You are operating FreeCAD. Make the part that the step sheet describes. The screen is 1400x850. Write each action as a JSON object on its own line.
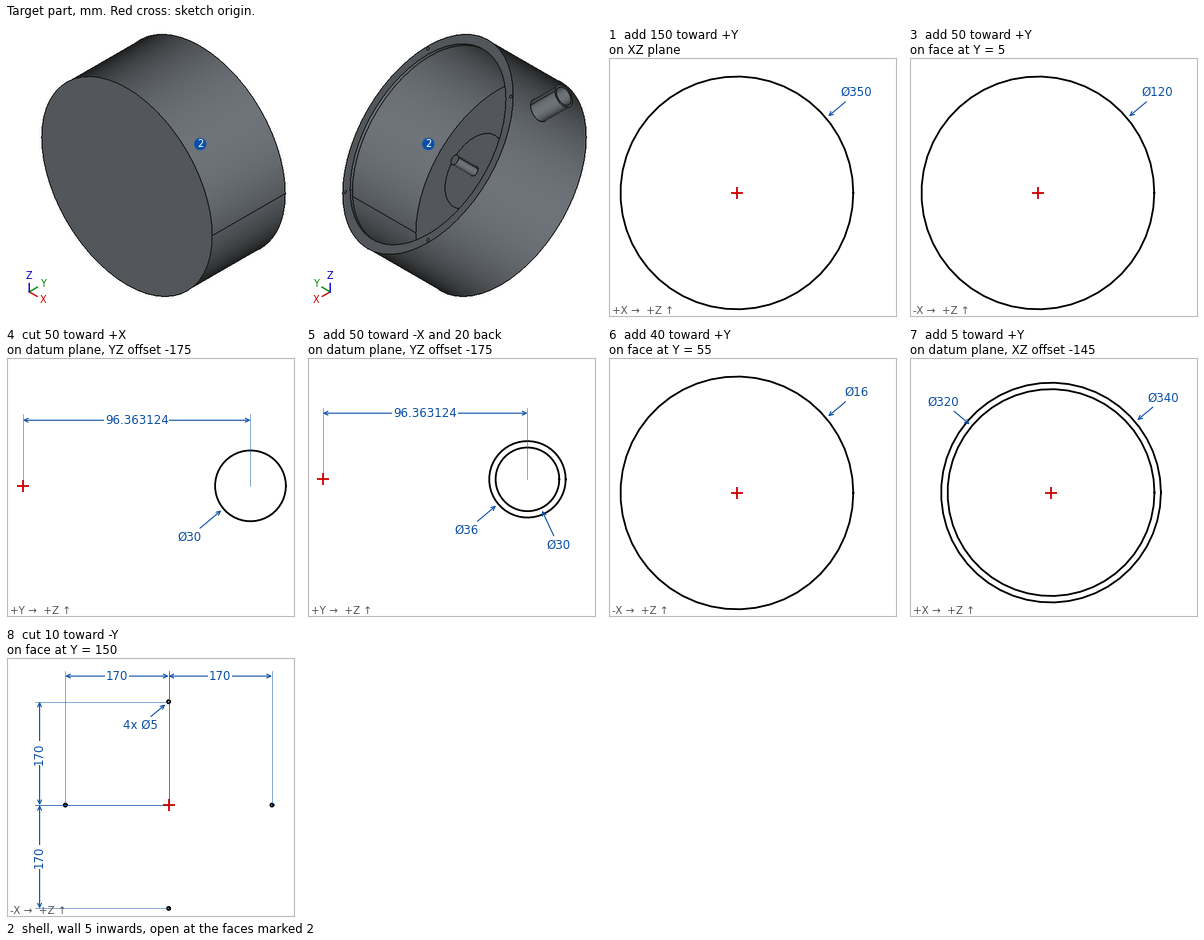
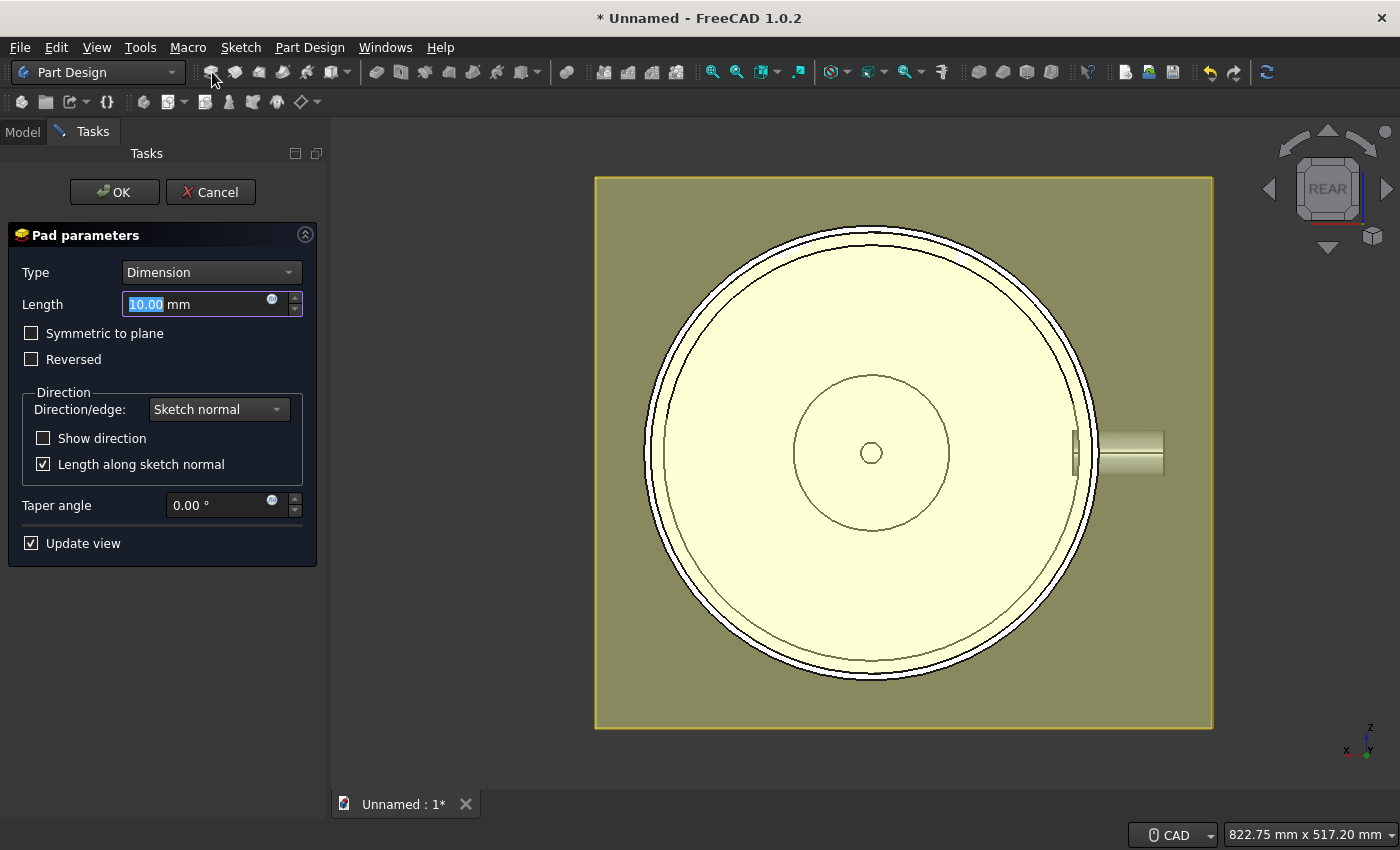
{"action": "type", "text": "5"}
{"action": "key", "text": "Tab"}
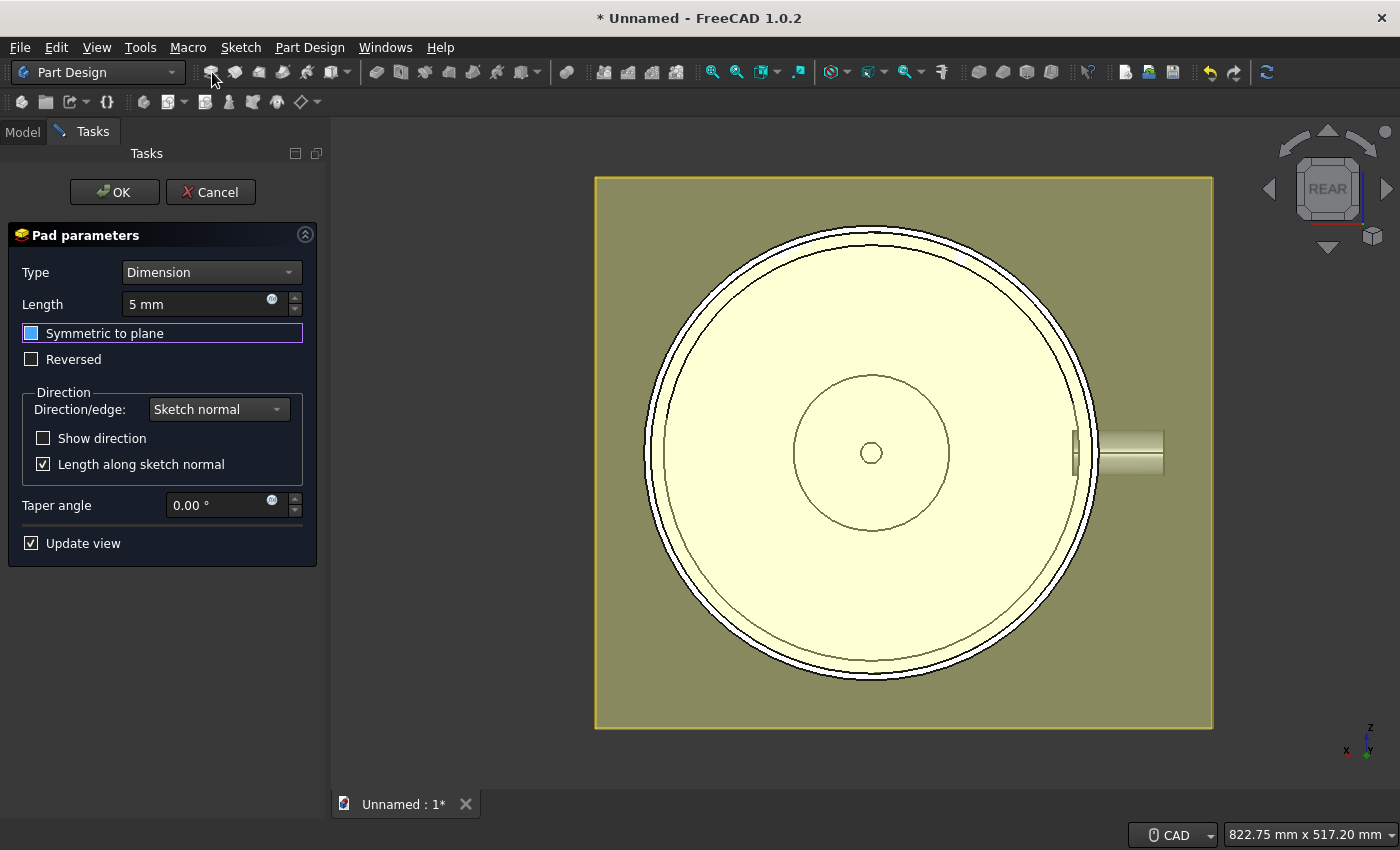
{"action": "left_click", "coordinate": [30, 359]}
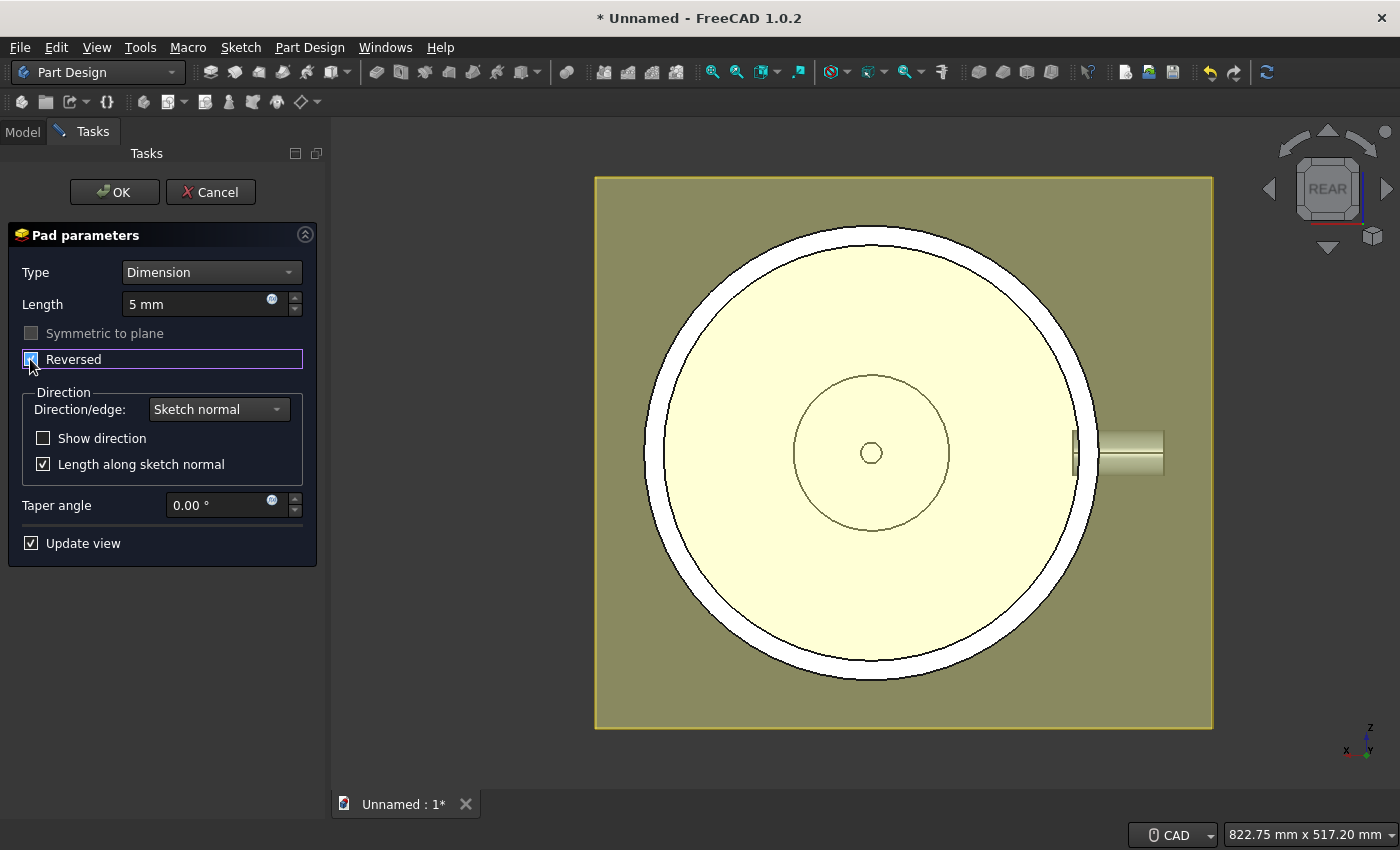
{"action": "left_click", "coordinate": [115, 192]}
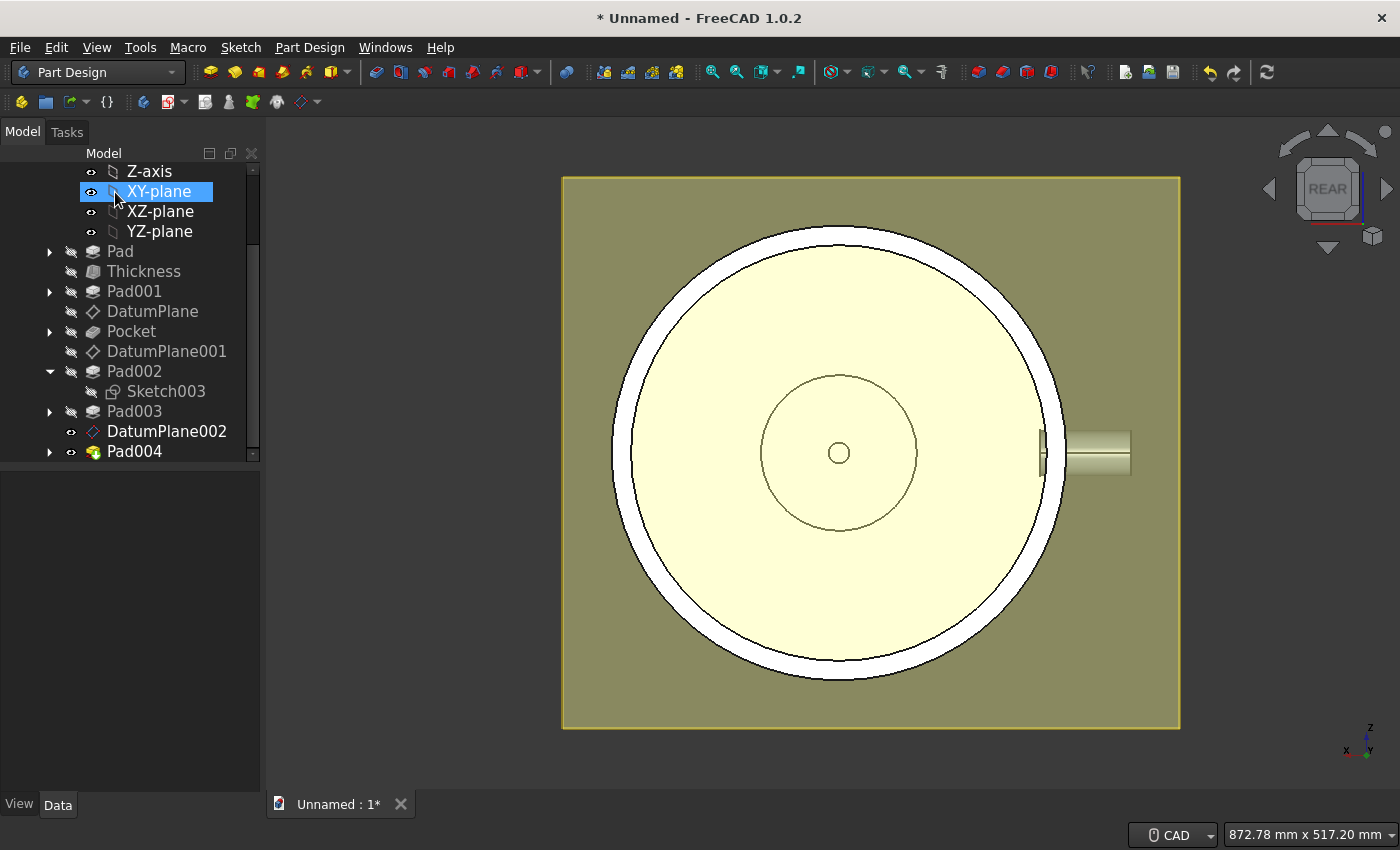
{"action": "left_click", "coordinate": [116, 432]}
{"action": "key", "text": "space"}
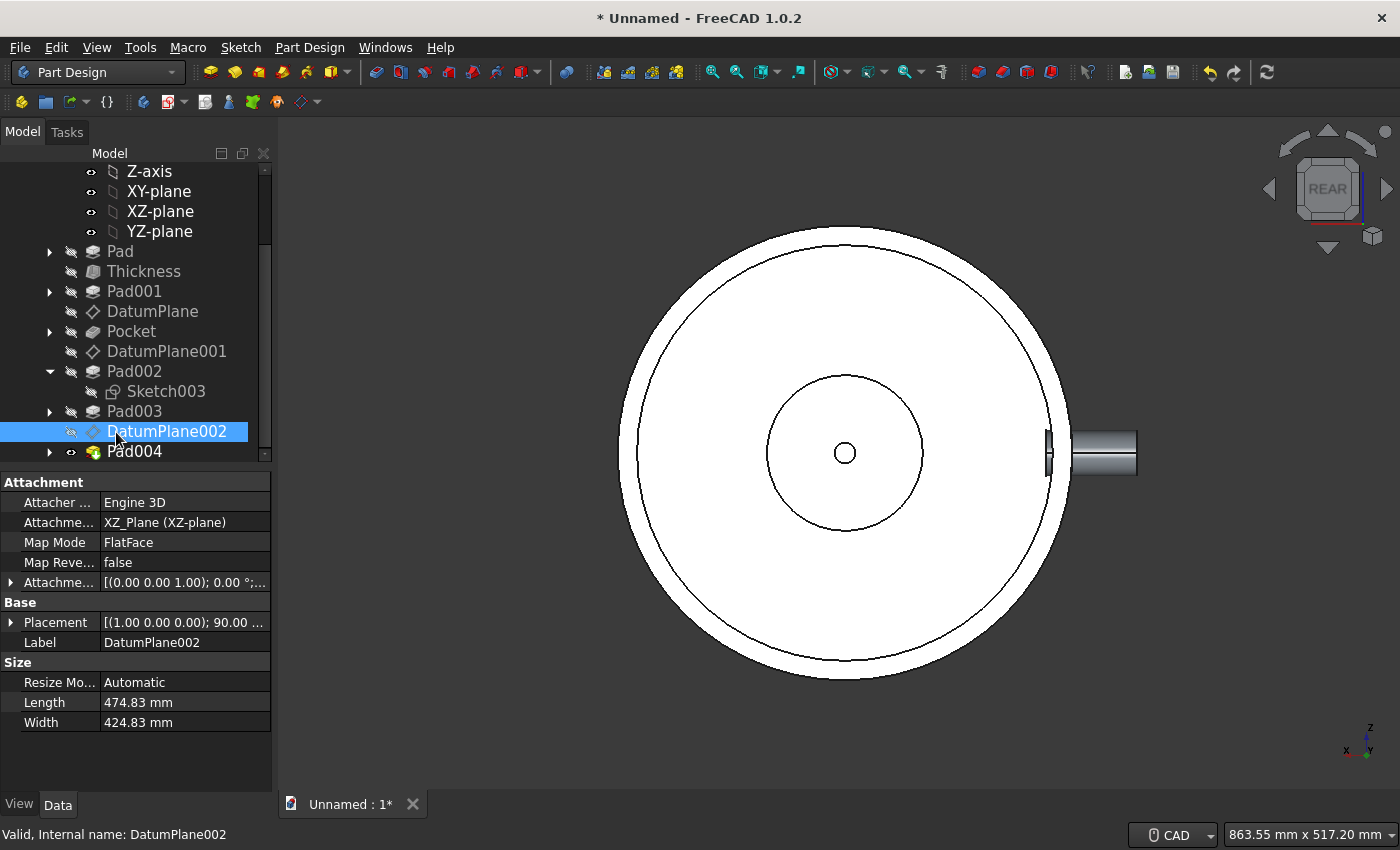
{"action": "left_click", "coordinate": [628, 412]}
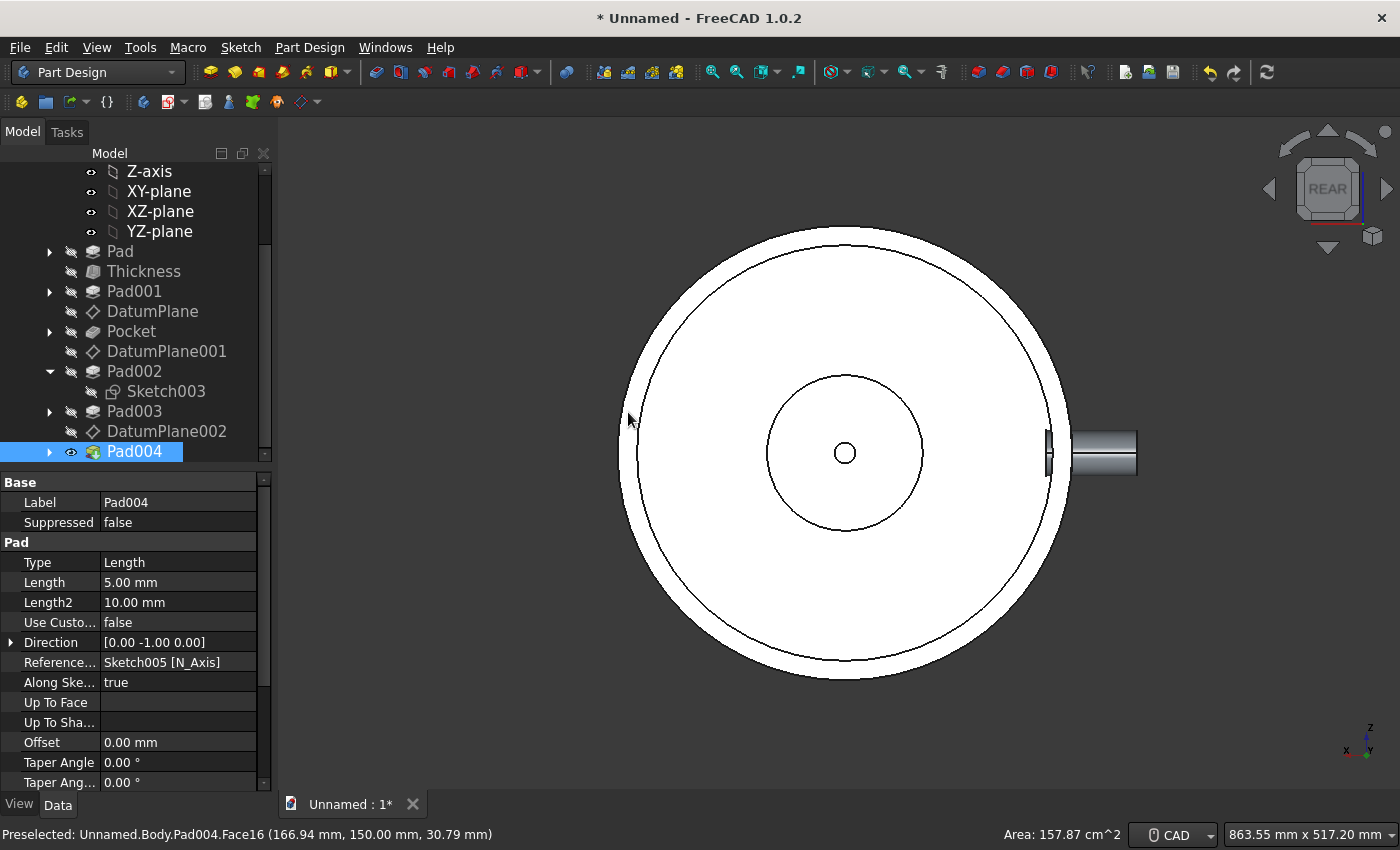
{"action": "left_click", "coordinate": [168, 102]}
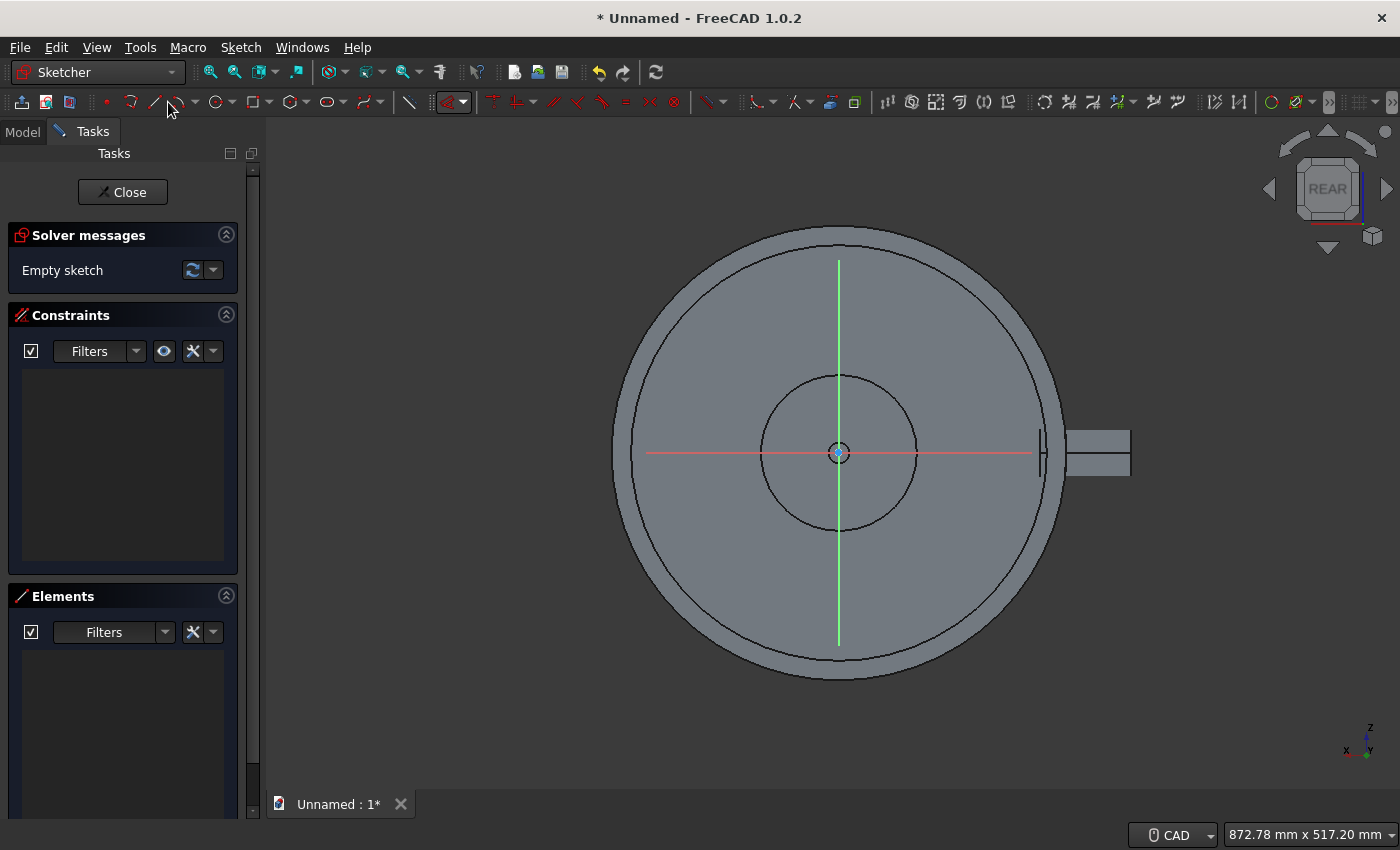
{"action": "left_click", "coordinate": [216, 102]}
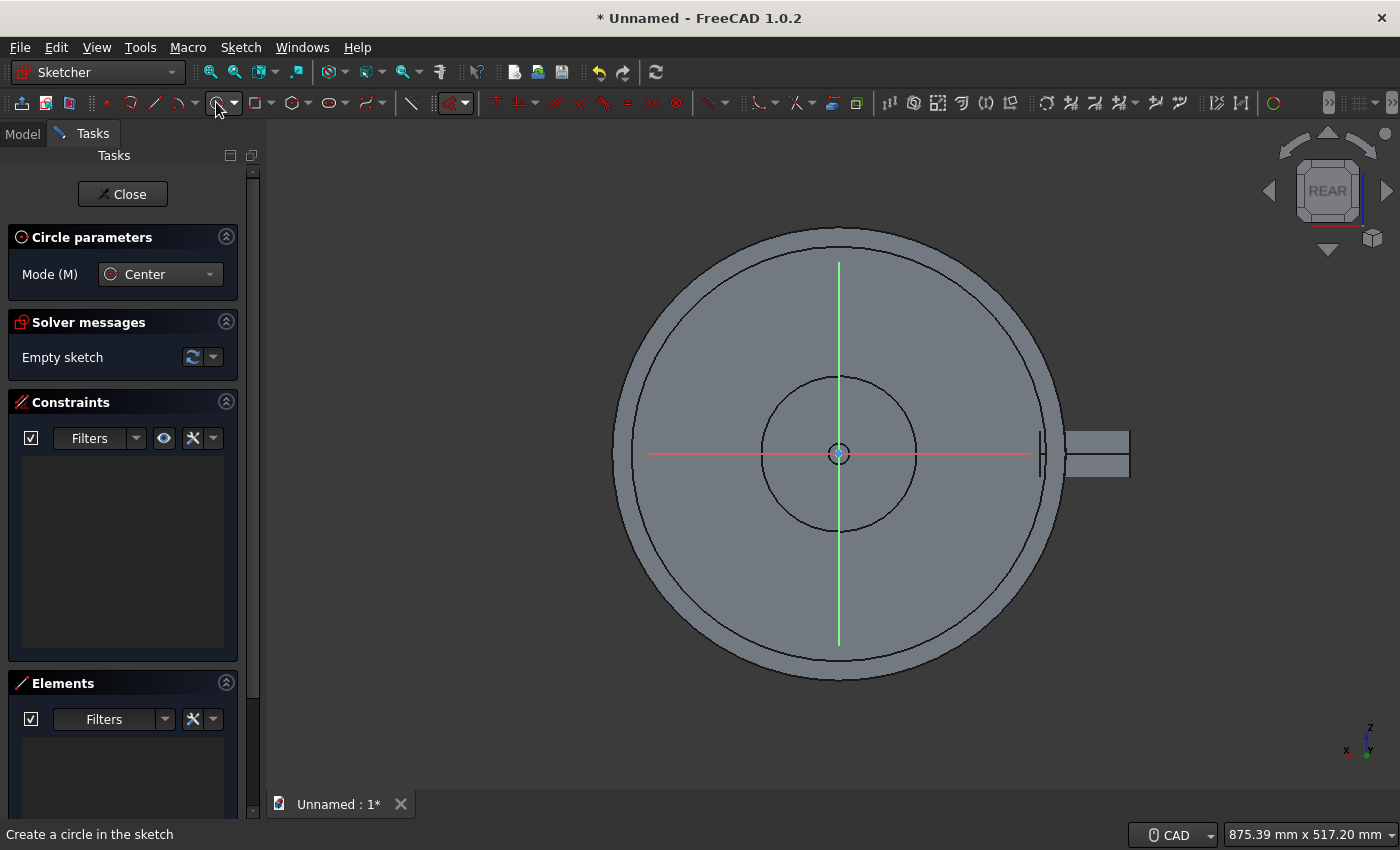
{"action": "scroll", "coordinate": [839, 234], "scroll_direction": "up", "scroll_amount": 10}